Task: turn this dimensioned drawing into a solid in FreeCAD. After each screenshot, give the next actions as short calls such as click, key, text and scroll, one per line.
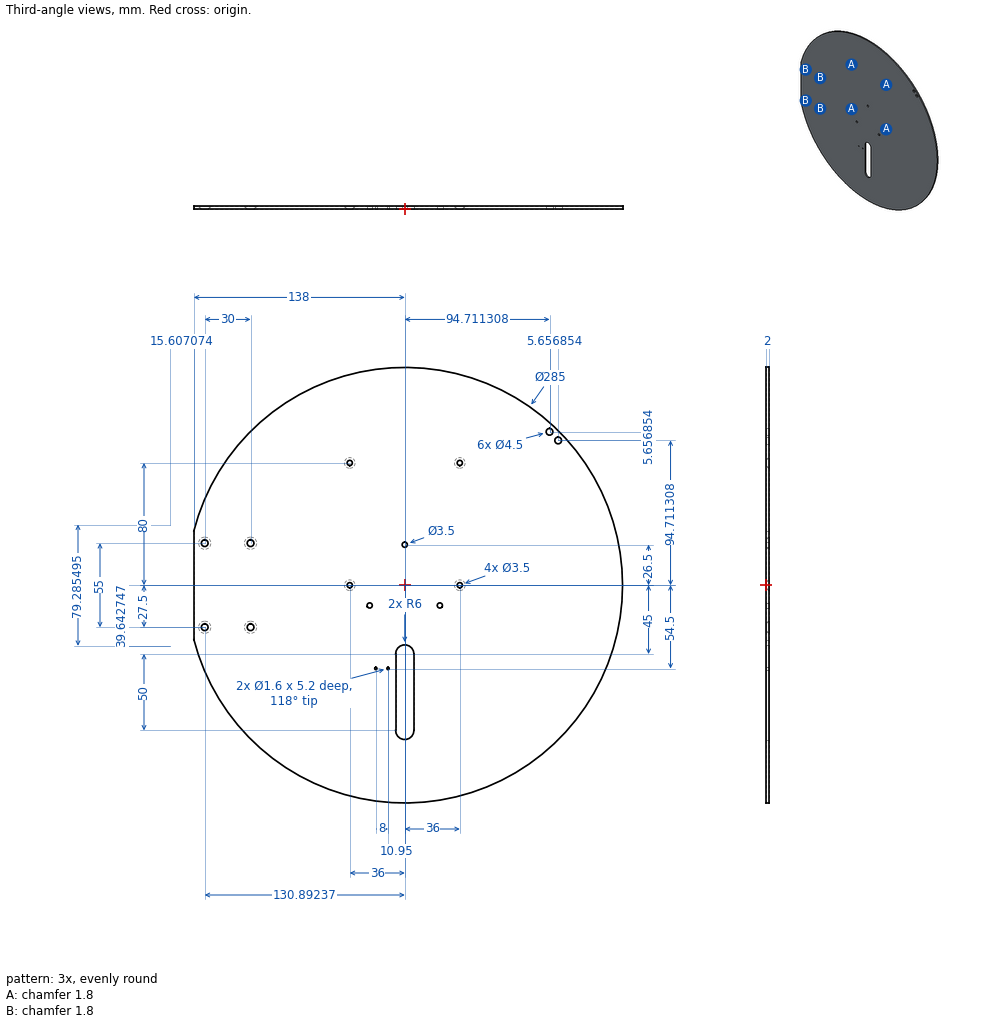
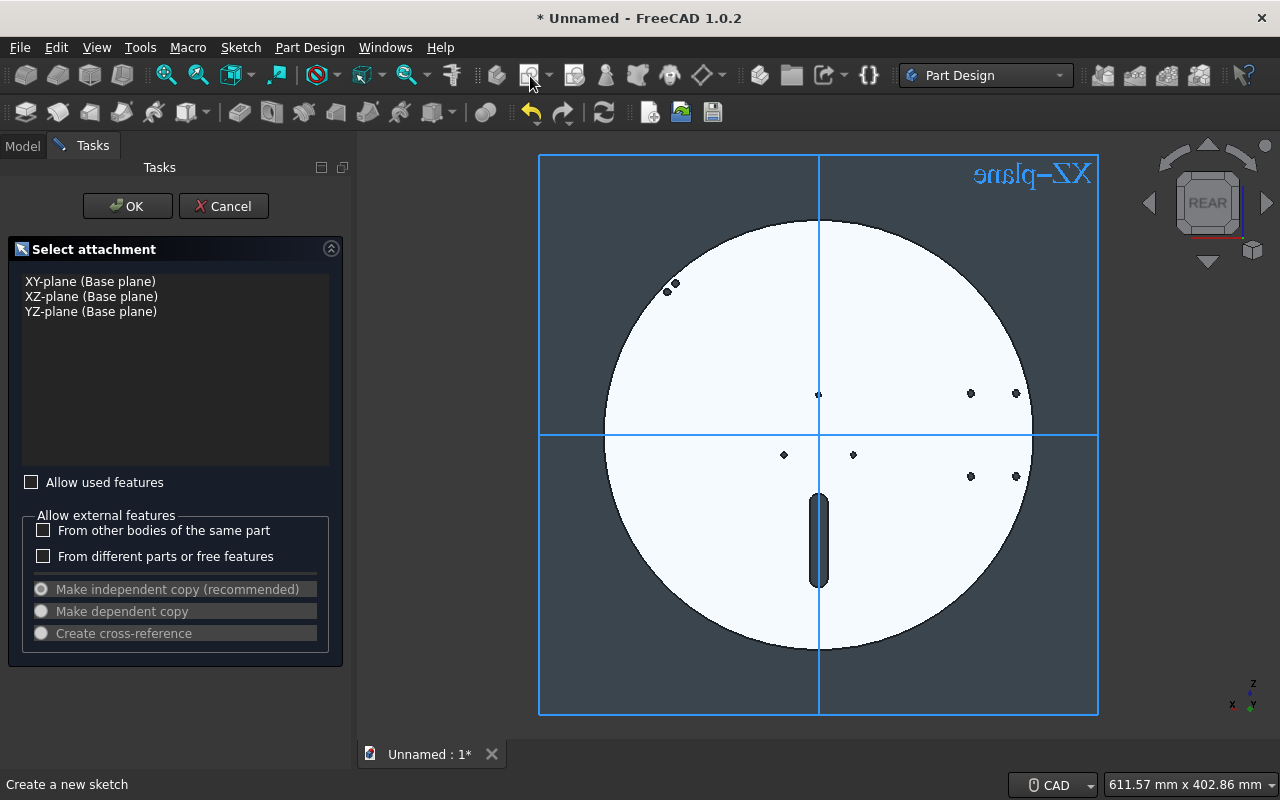
click(82, 296)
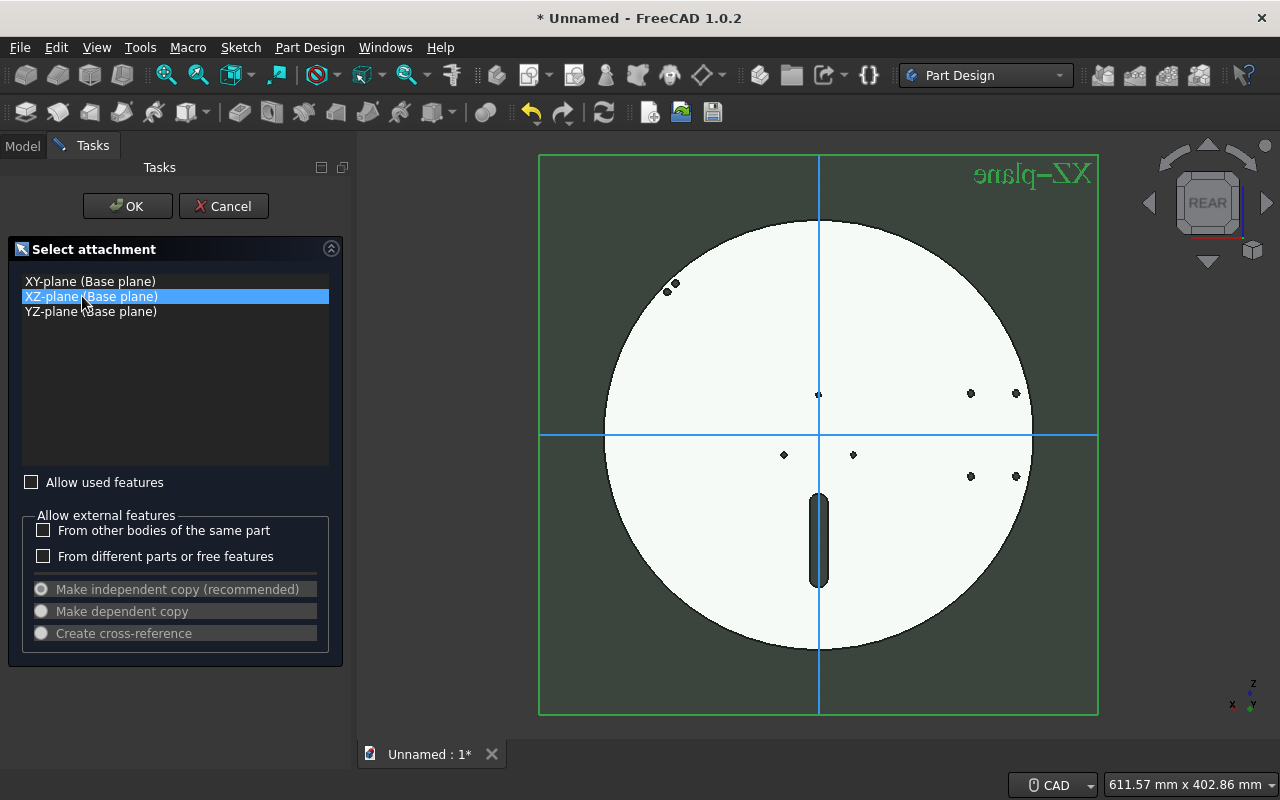
click(128, 206)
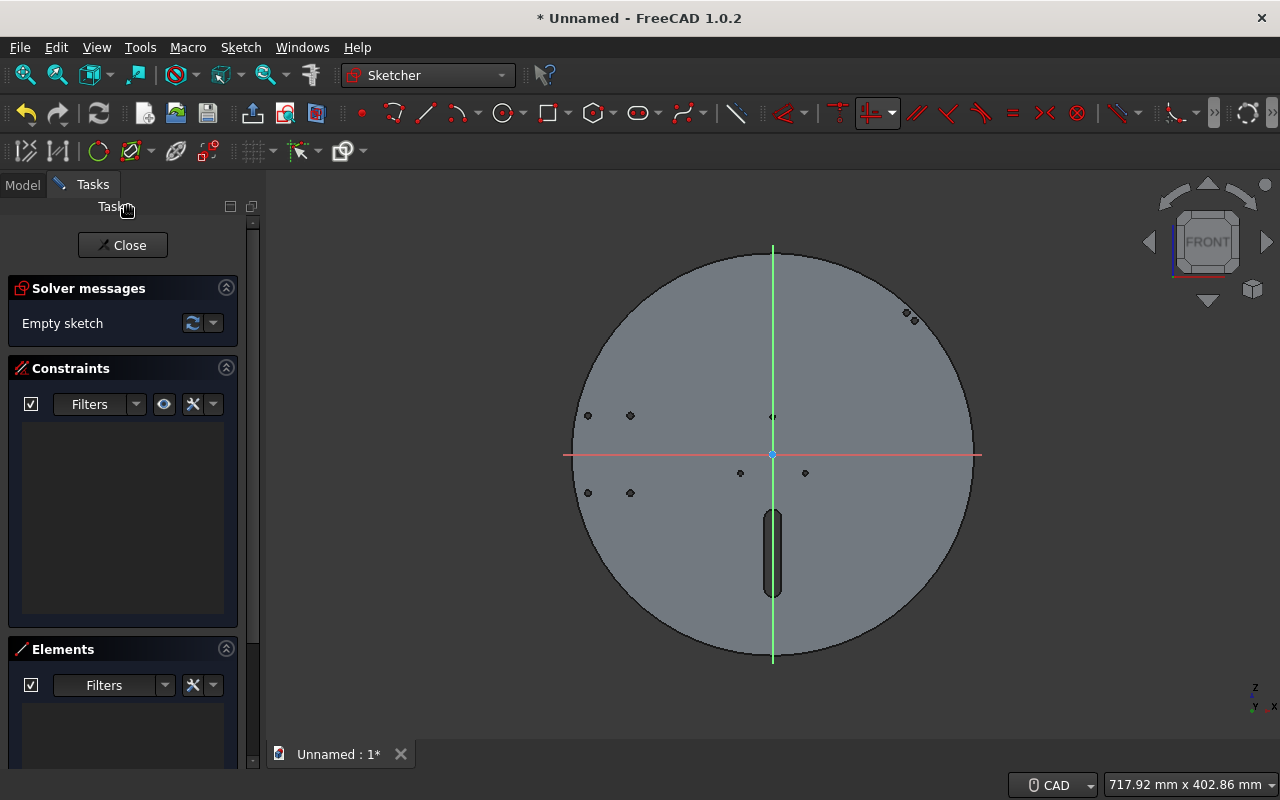
scroll(802, 374, up, 6)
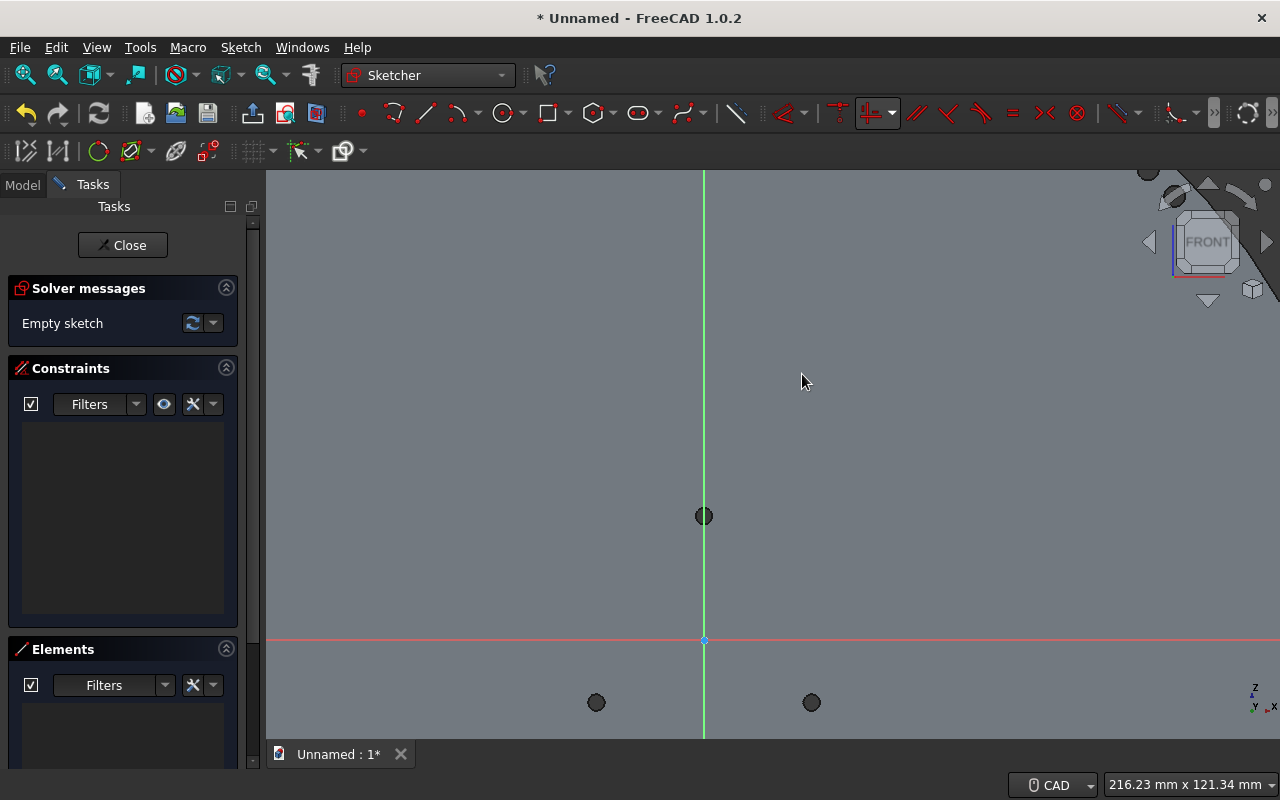
key(g)
key(c)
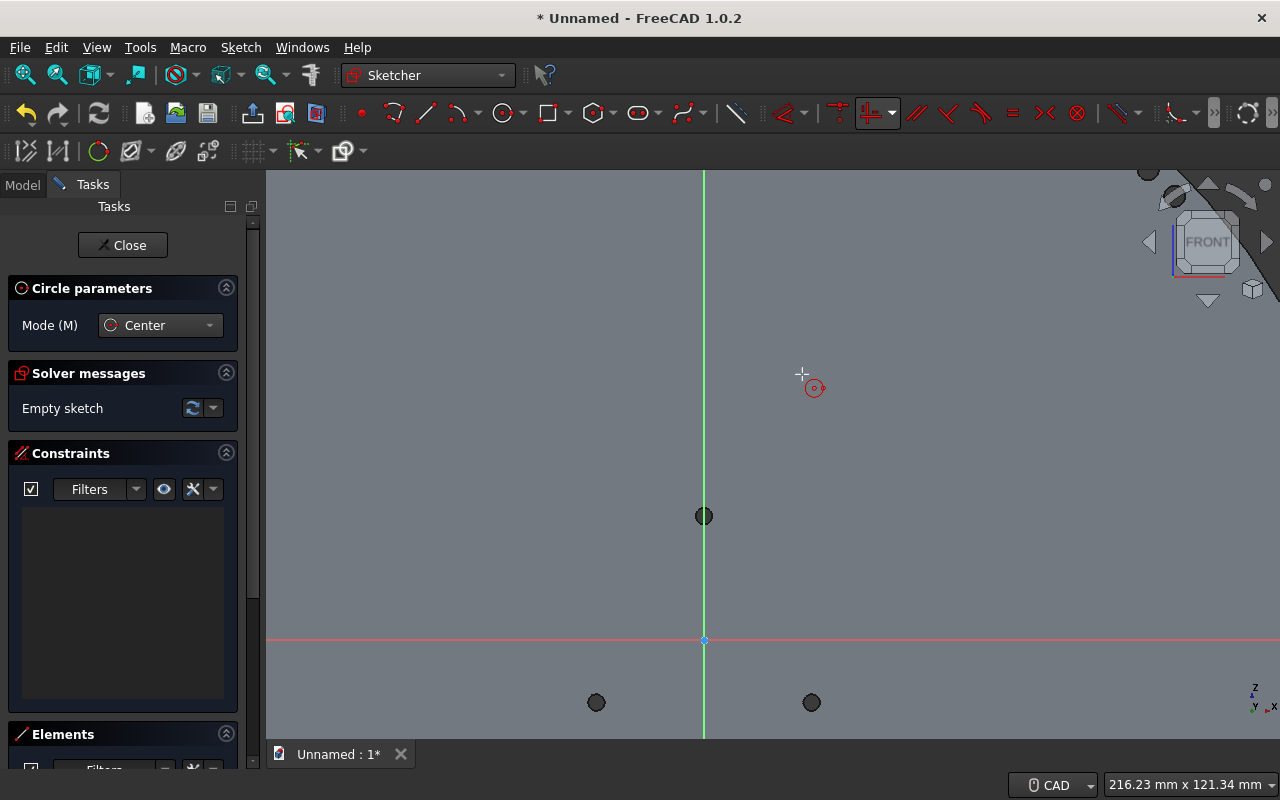
scroll(873, 640, up, 6)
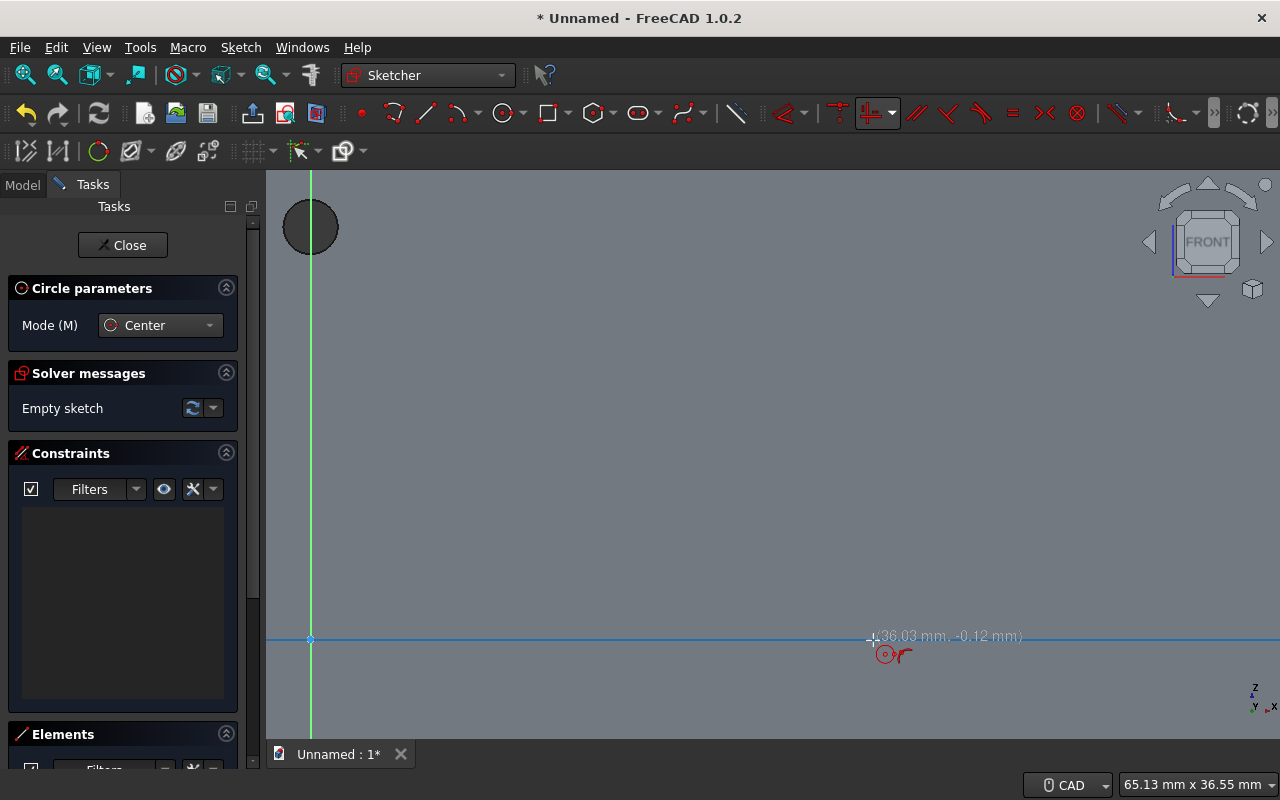
click(871, 640)
click(890, 620)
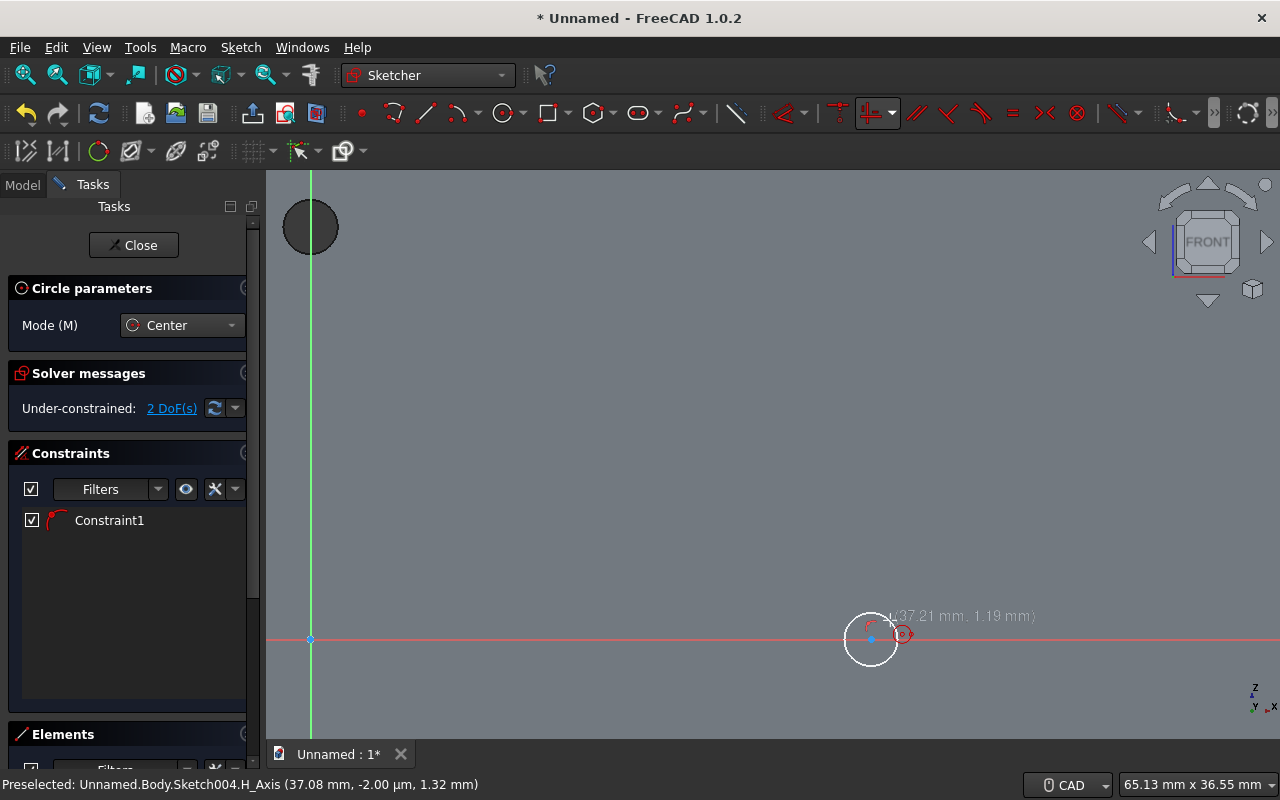
scroll(874, 643, down, 6)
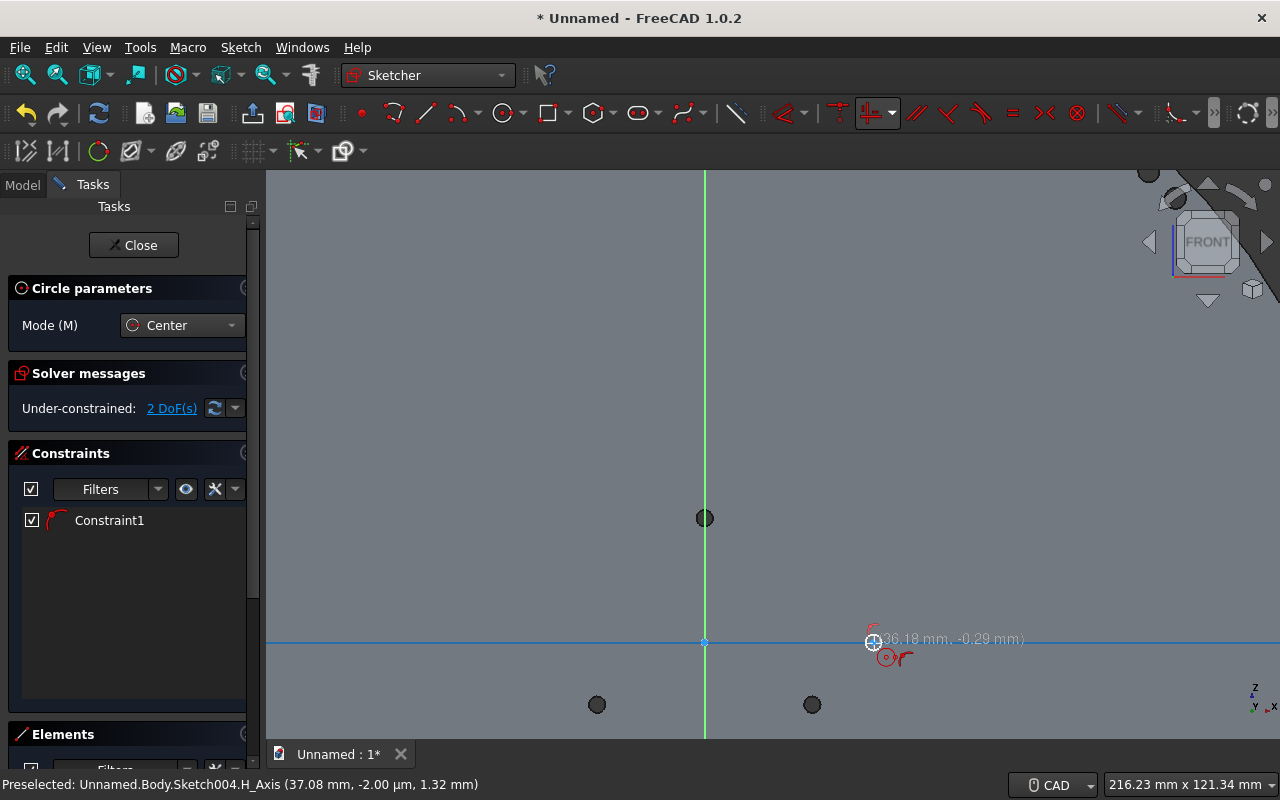
scroll(536, 643, up, 6)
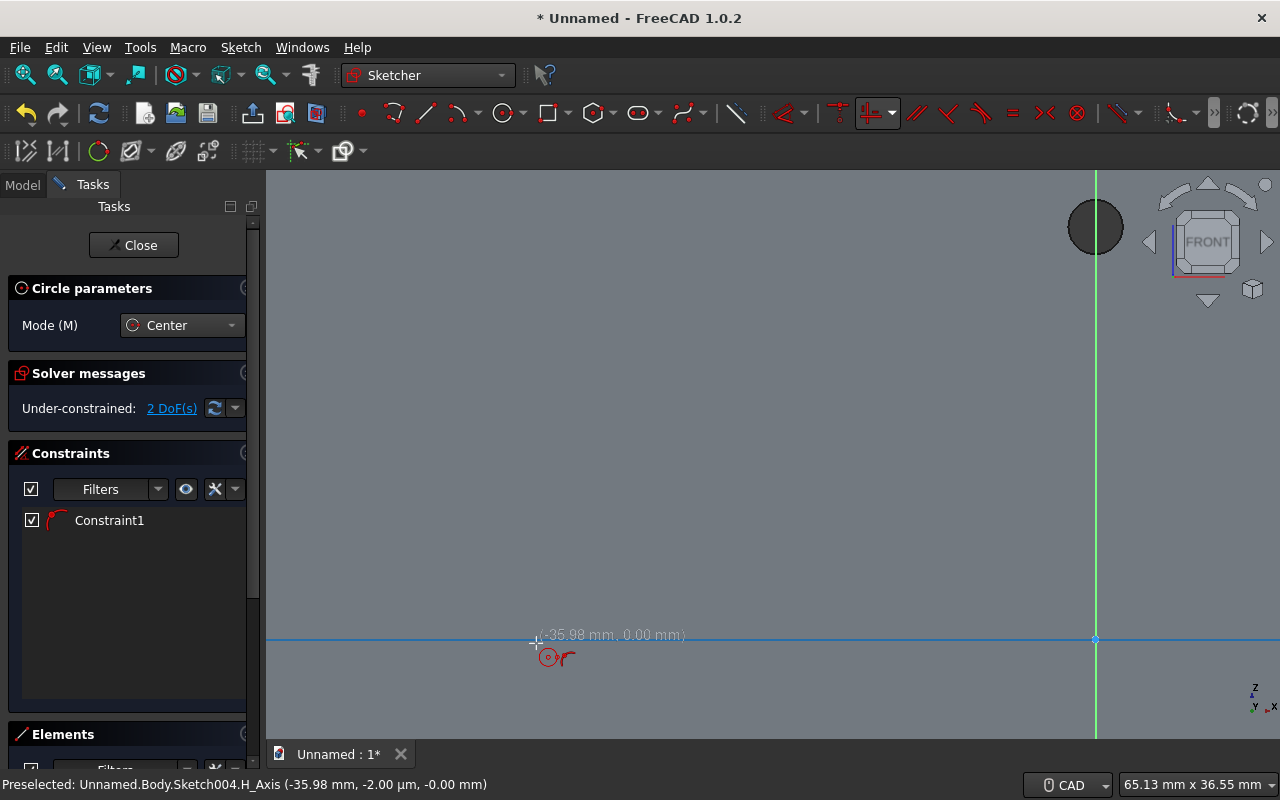
click(535, 640)
click(554, 620)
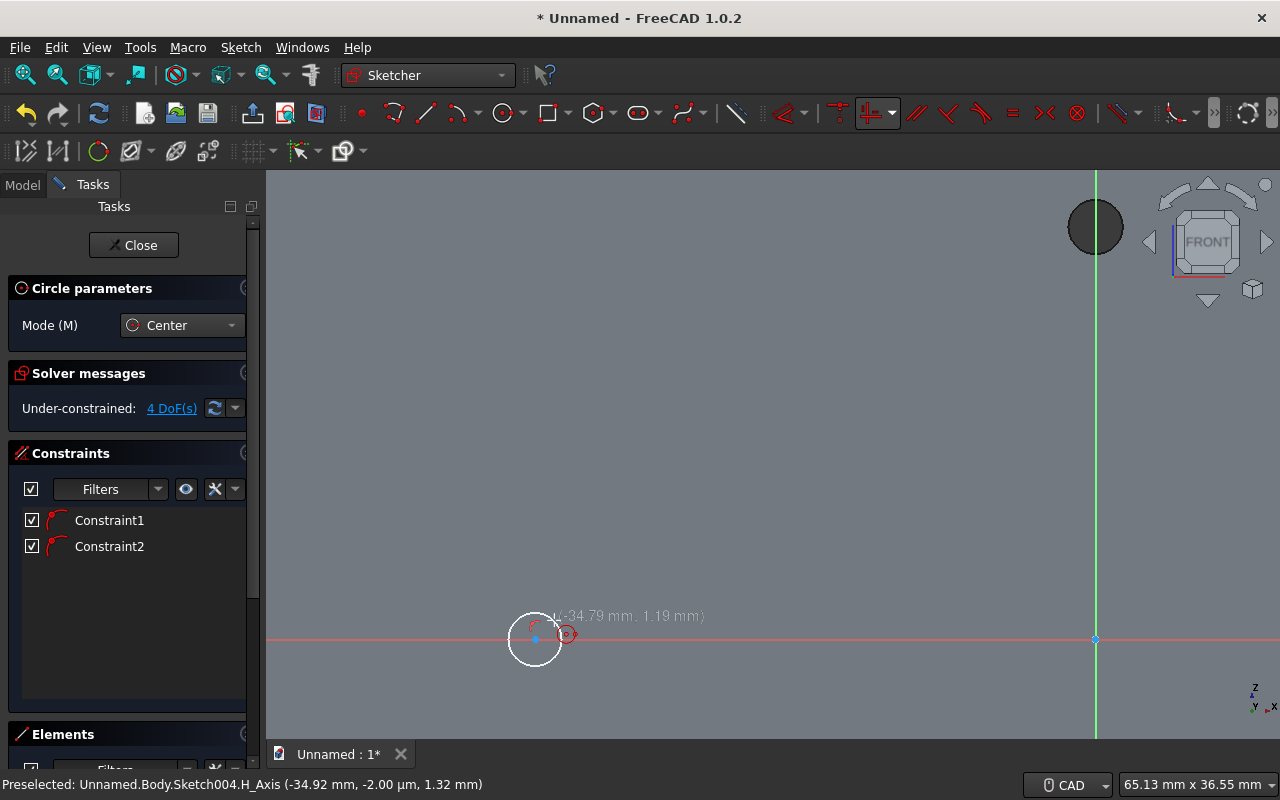
scroll(536, 643, down, 6)